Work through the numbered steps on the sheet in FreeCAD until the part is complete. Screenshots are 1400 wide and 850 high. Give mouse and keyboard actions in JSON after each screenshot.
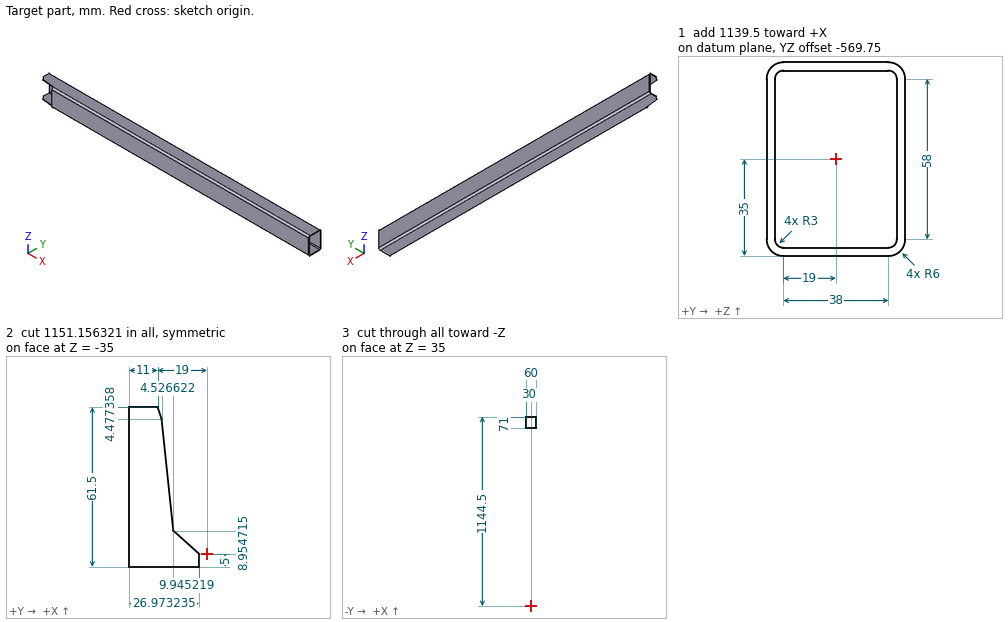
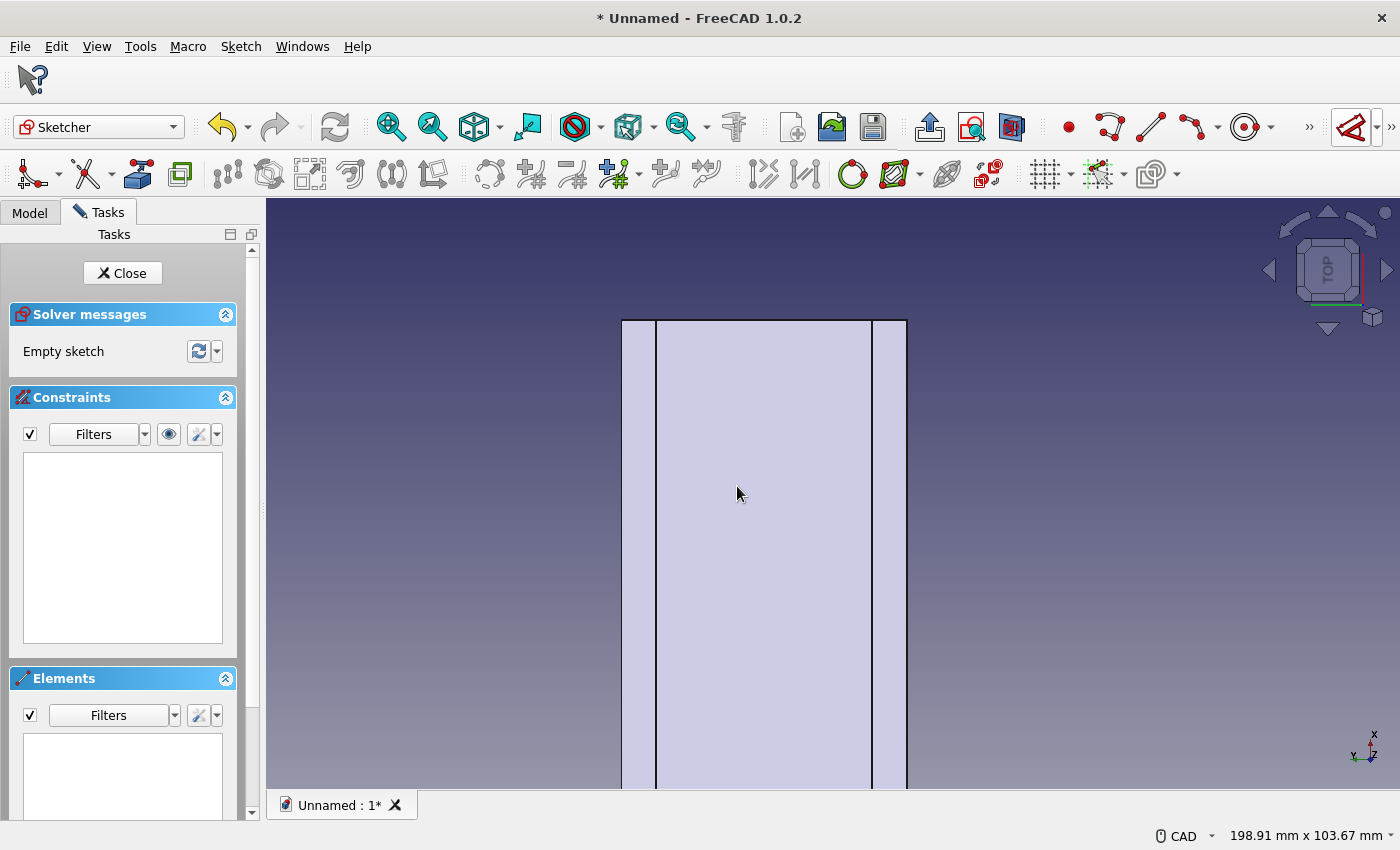
{"action": "key", "text": "g r"}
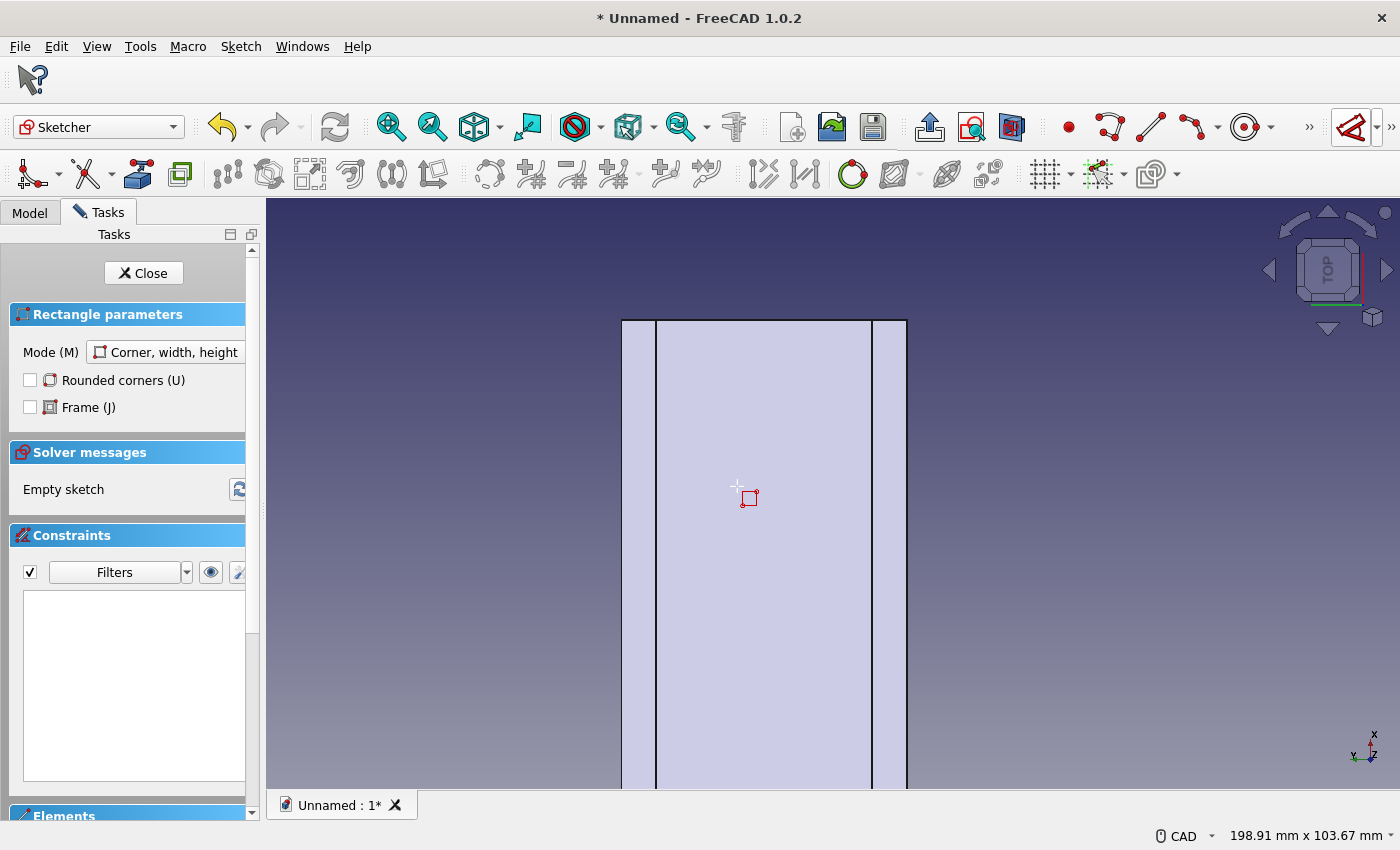
{"action": "left_click", "coordinate": [593, 291]}
{"action": "left_click", "coordinate": [935, 696]}
{"action": "key", "text": "Escape"}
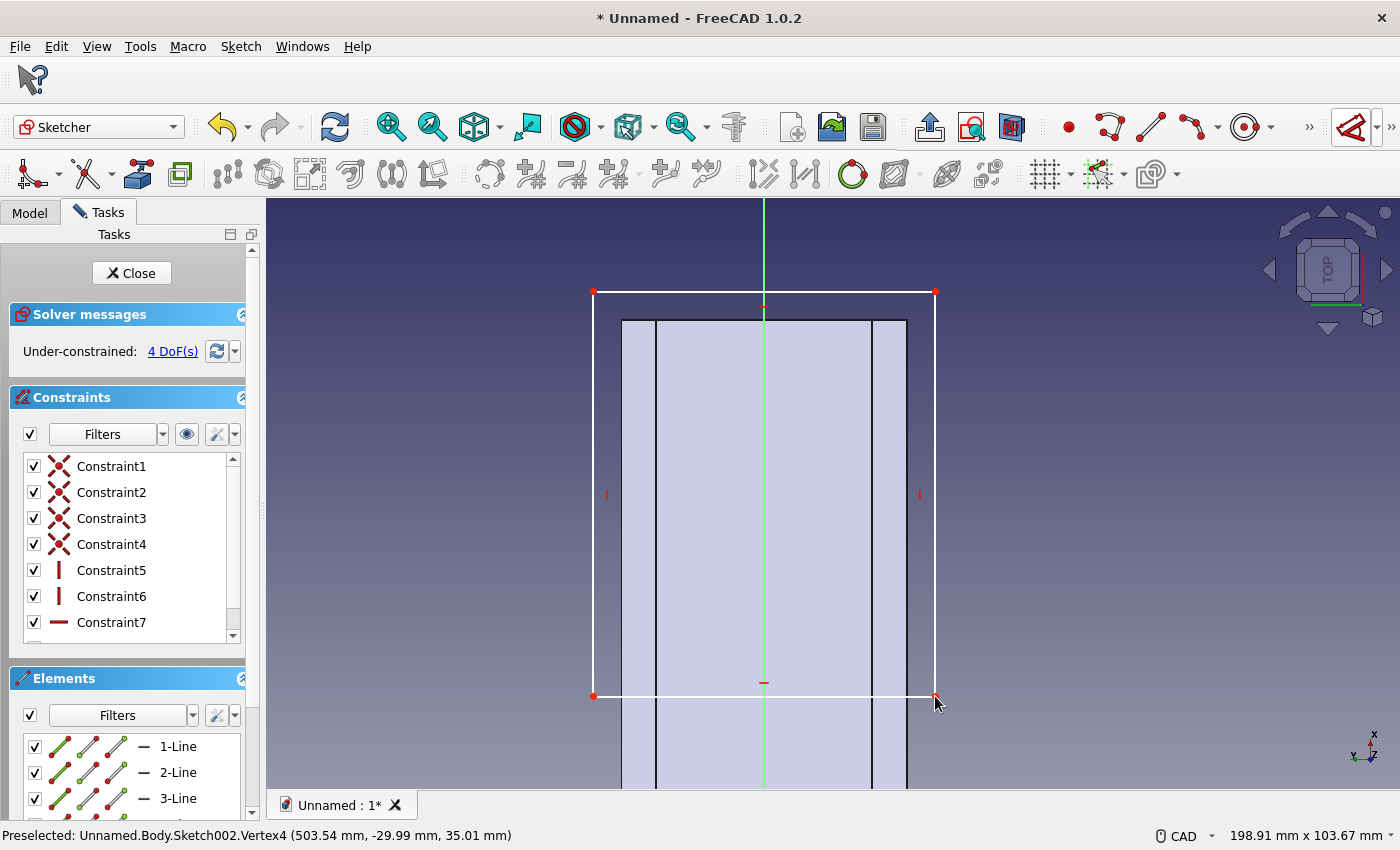
{"action": "left_click", "coordinate": [593, 414]}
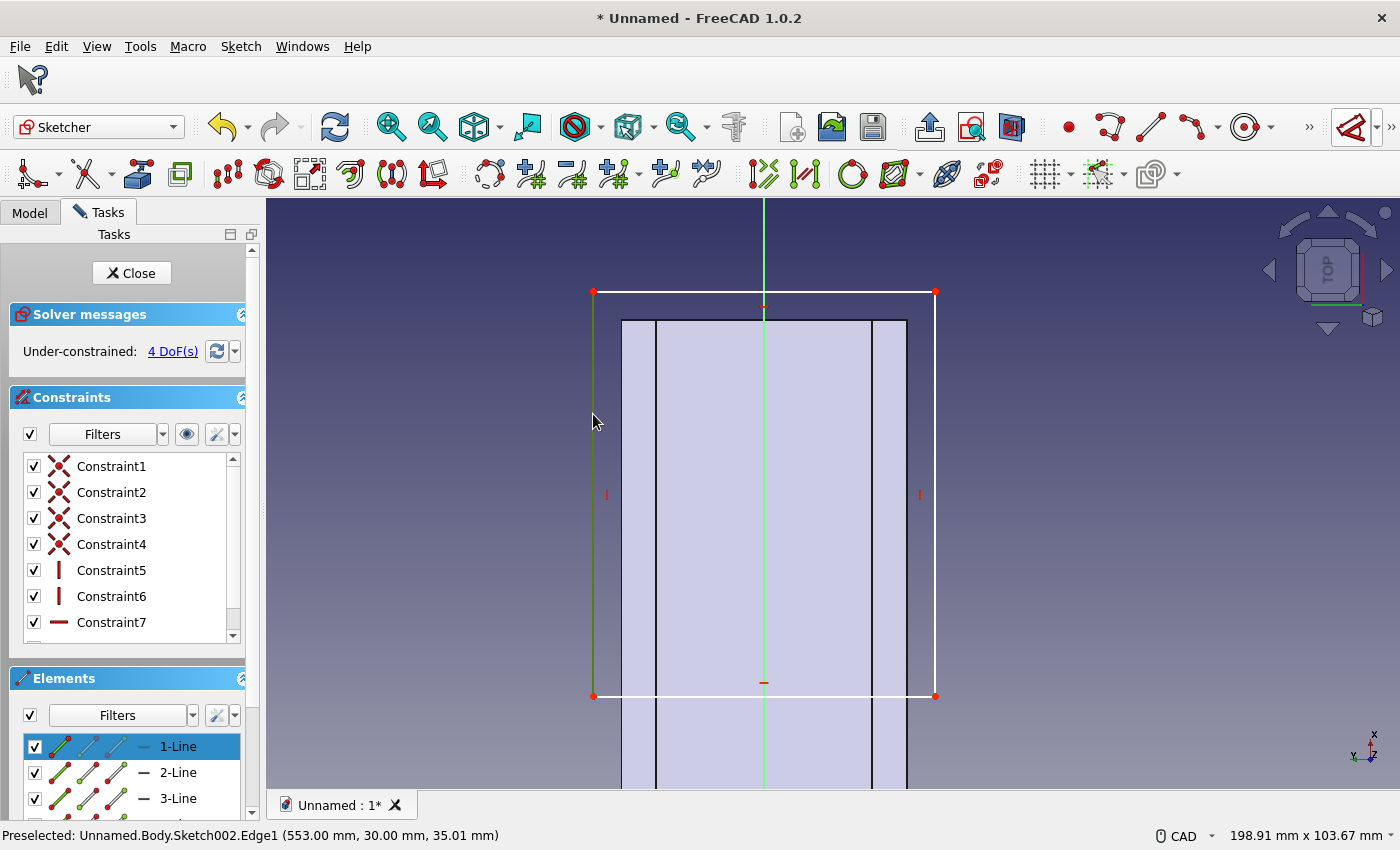
{"action": "key", "text": "i"}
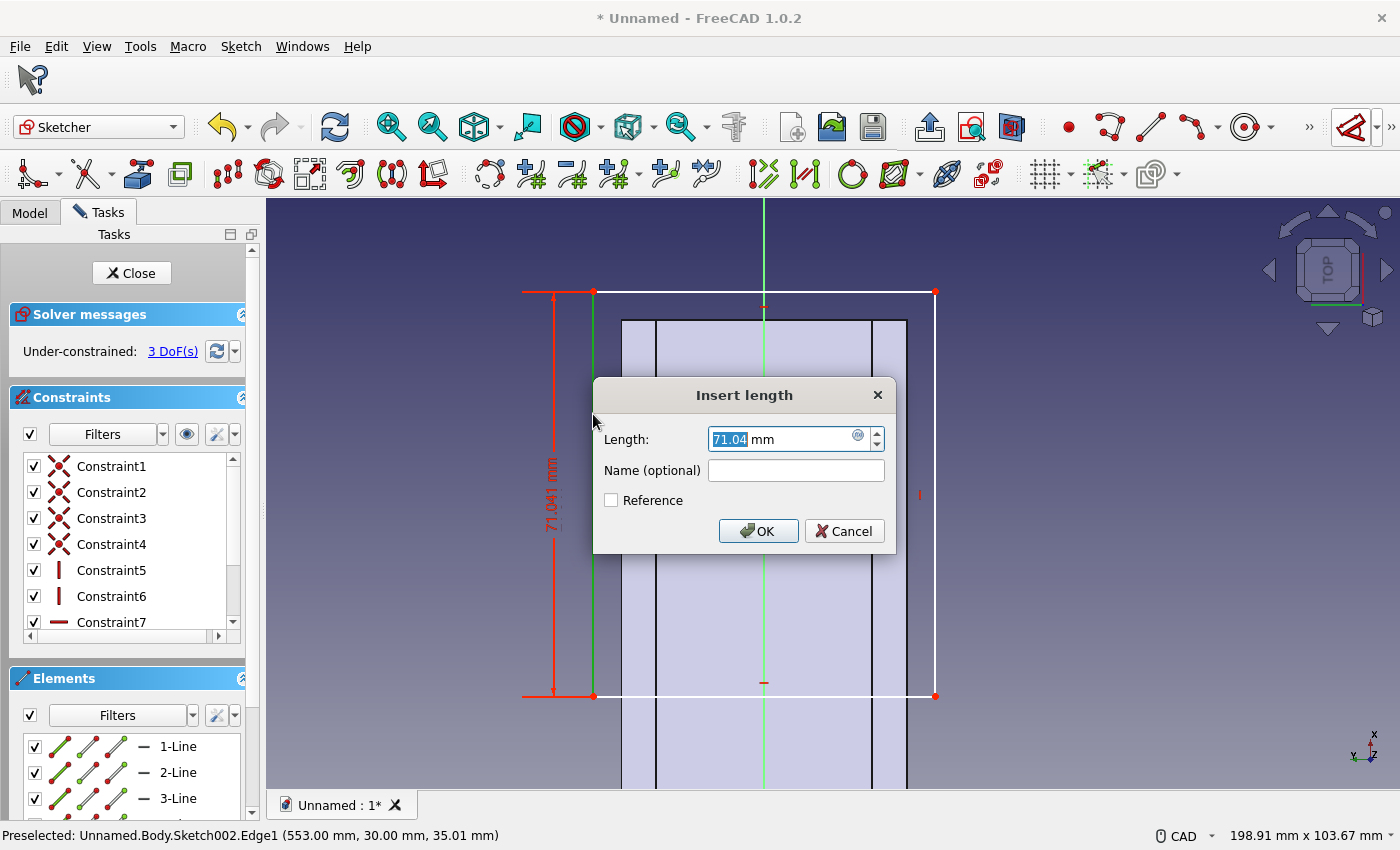
{"action": "type", "text": "71"}
{"action": "key", "text": "Return"}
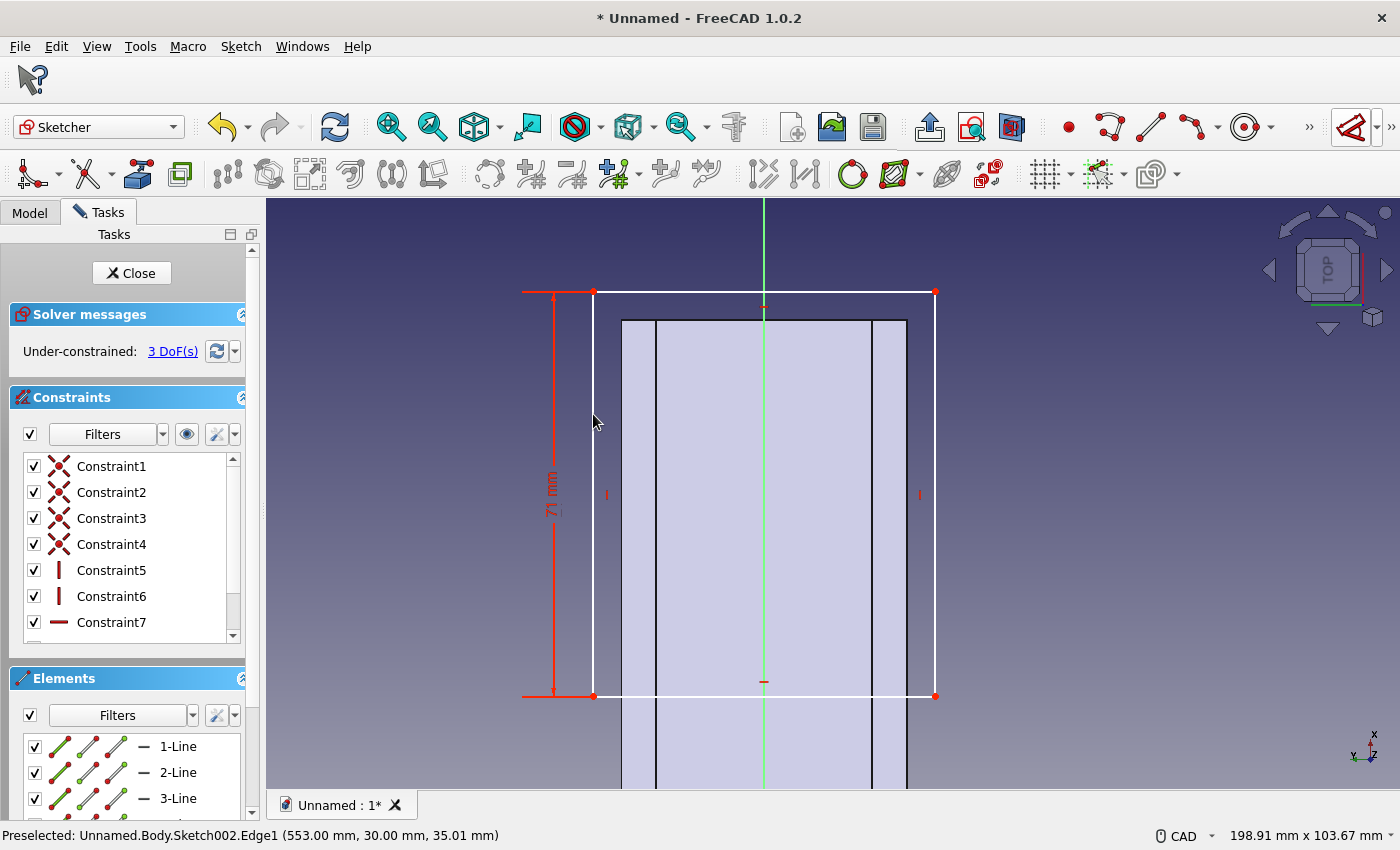
{"action": "left_click", "coordinate": [696, 697]}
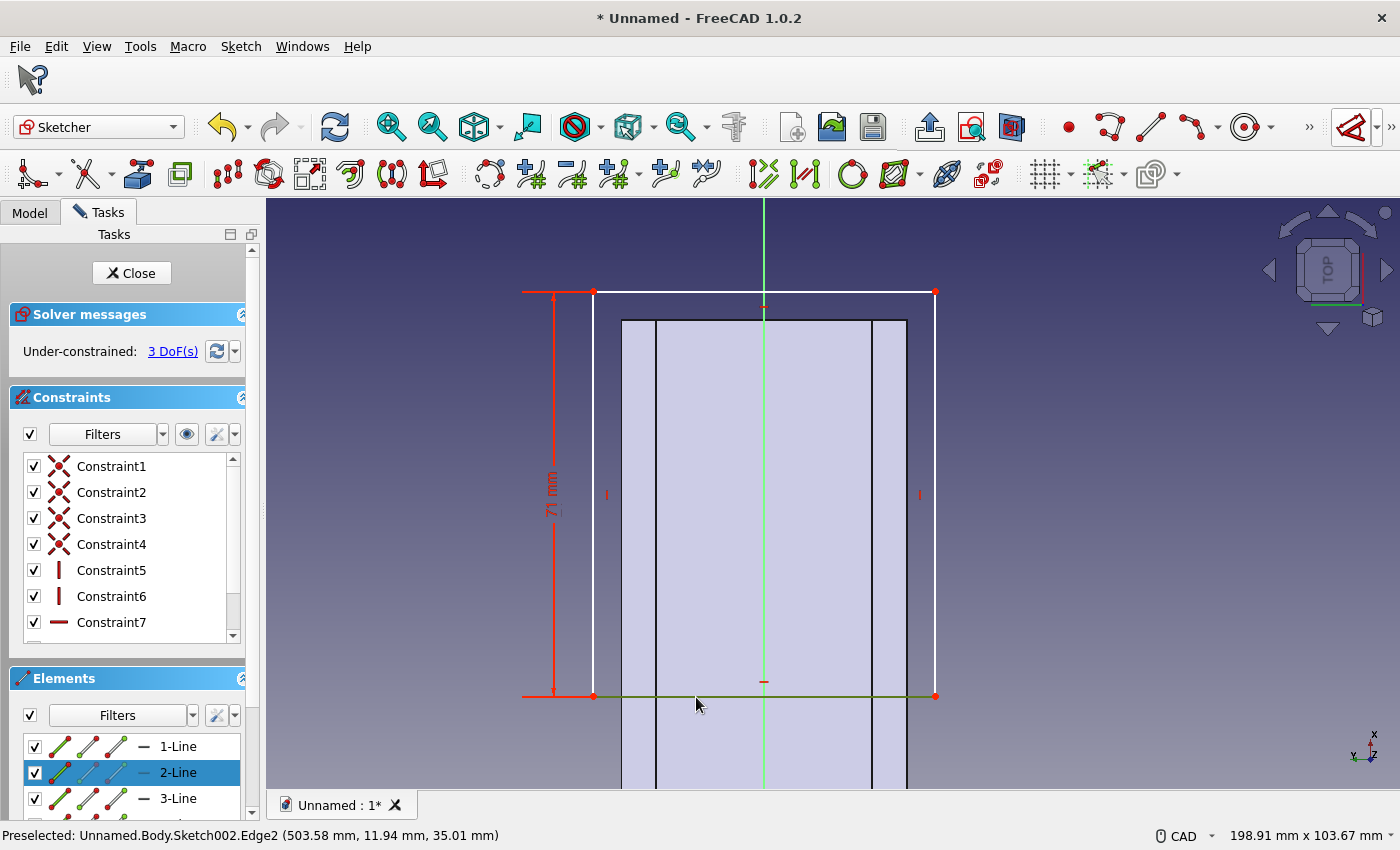
{"action": "key", "text": "l"}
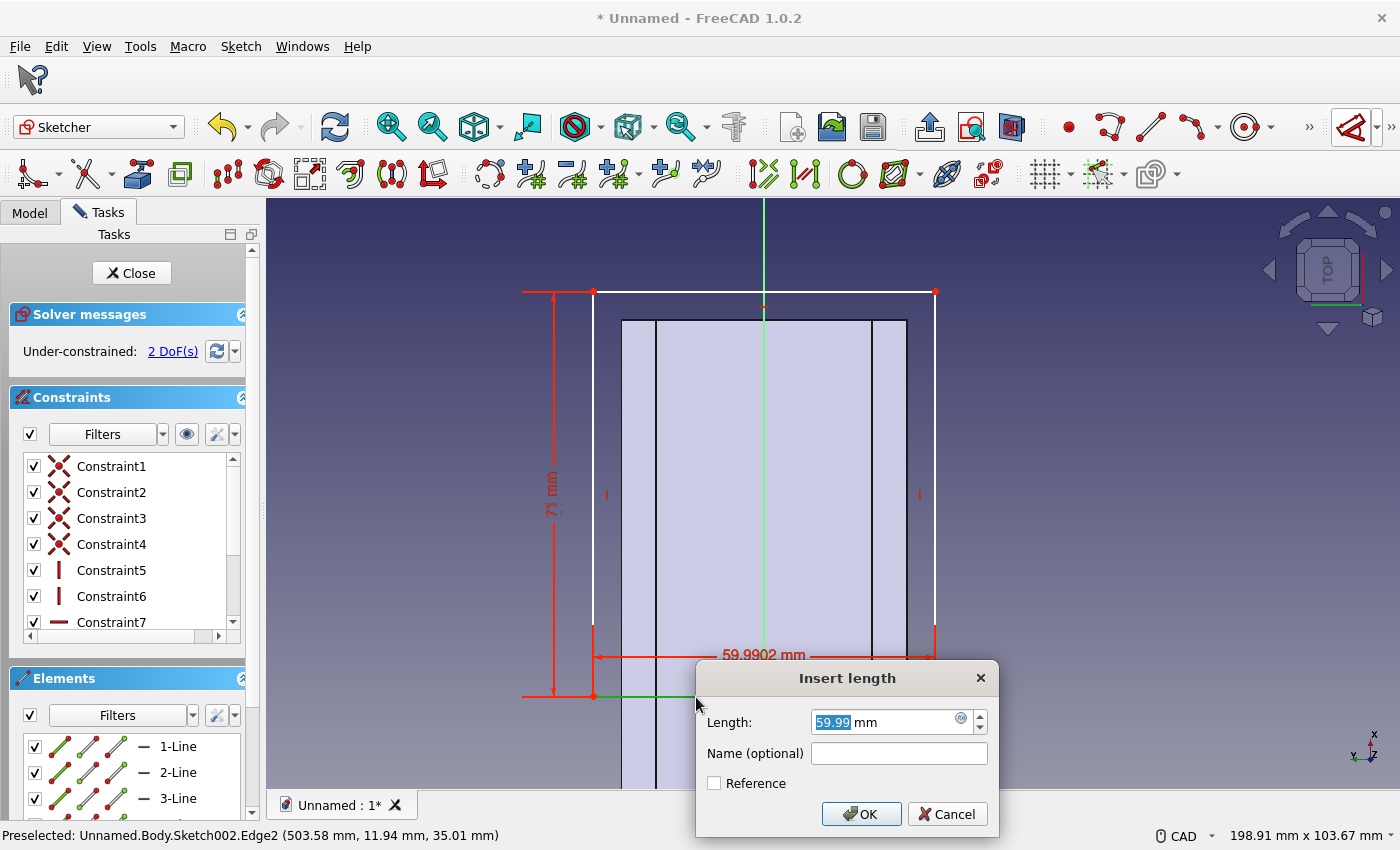
{"action": "type", "text": "60"}
{"action": "key", "text": "Return"}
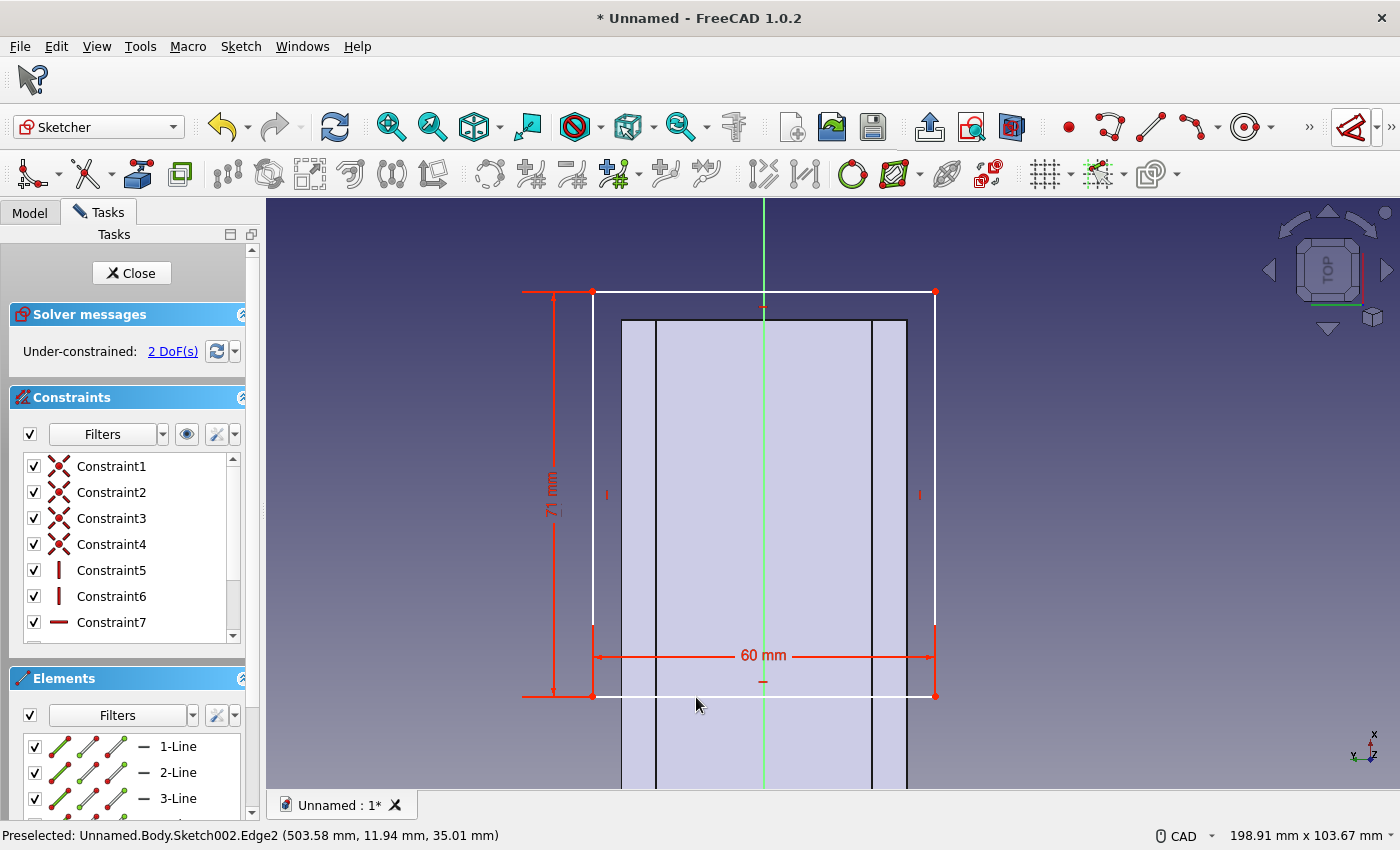
{"action": "left_click", "coordinate": [593, 292]}